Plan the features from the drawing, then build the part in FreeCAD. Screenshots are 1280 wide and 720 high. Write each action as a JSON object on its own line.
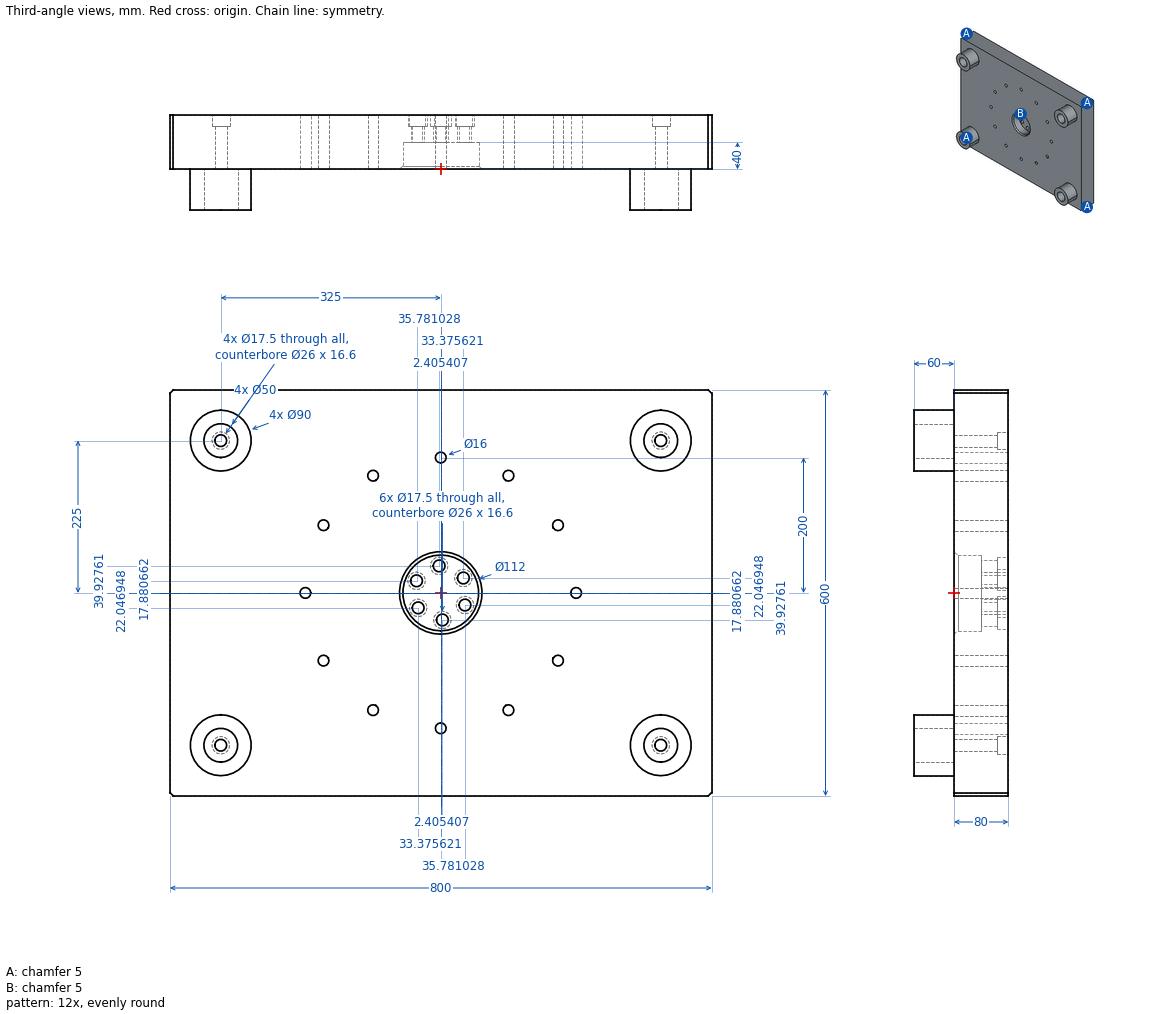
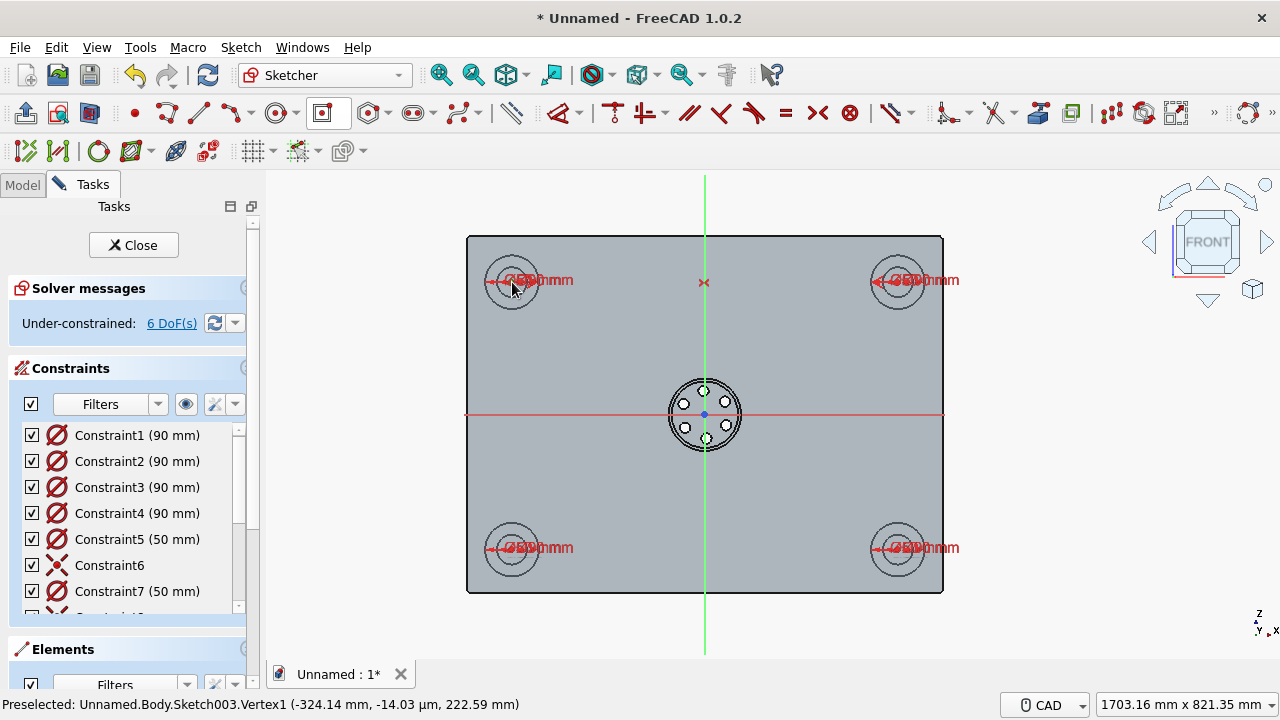
{"action": "left_click", "coordinate": [512, 550]}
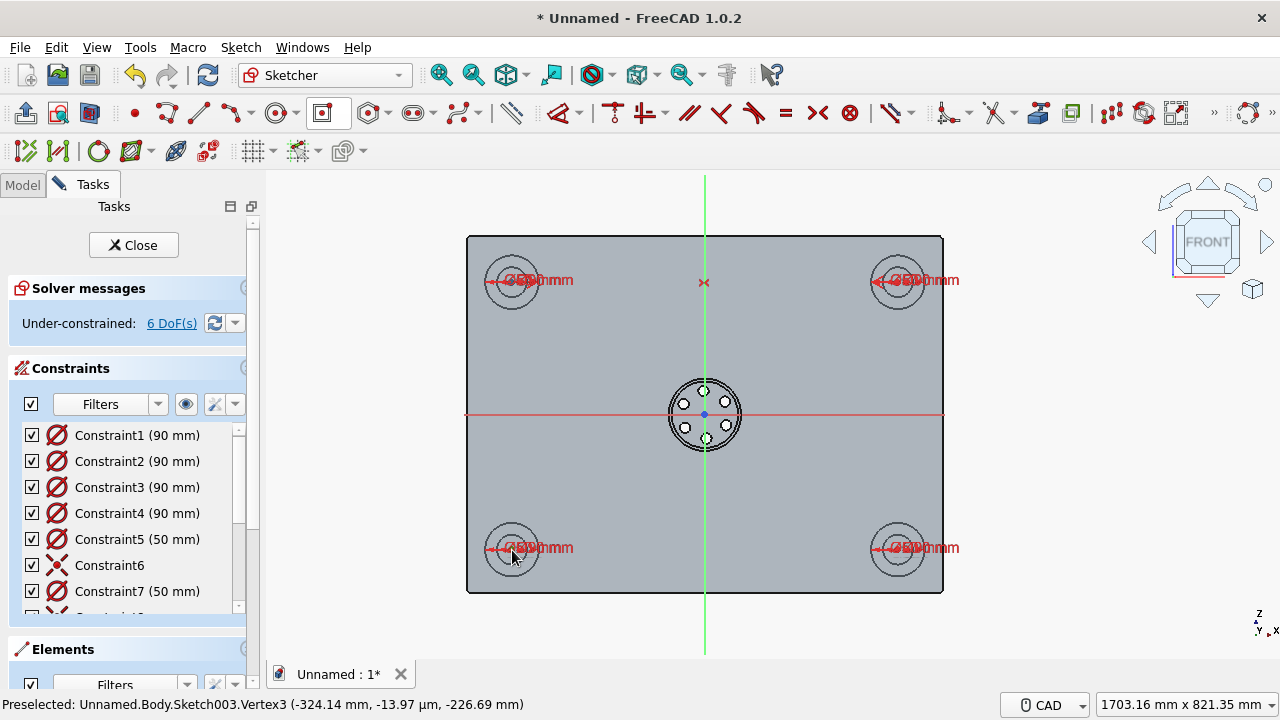
{"action": "left_click", "coordinate": [470, 415]}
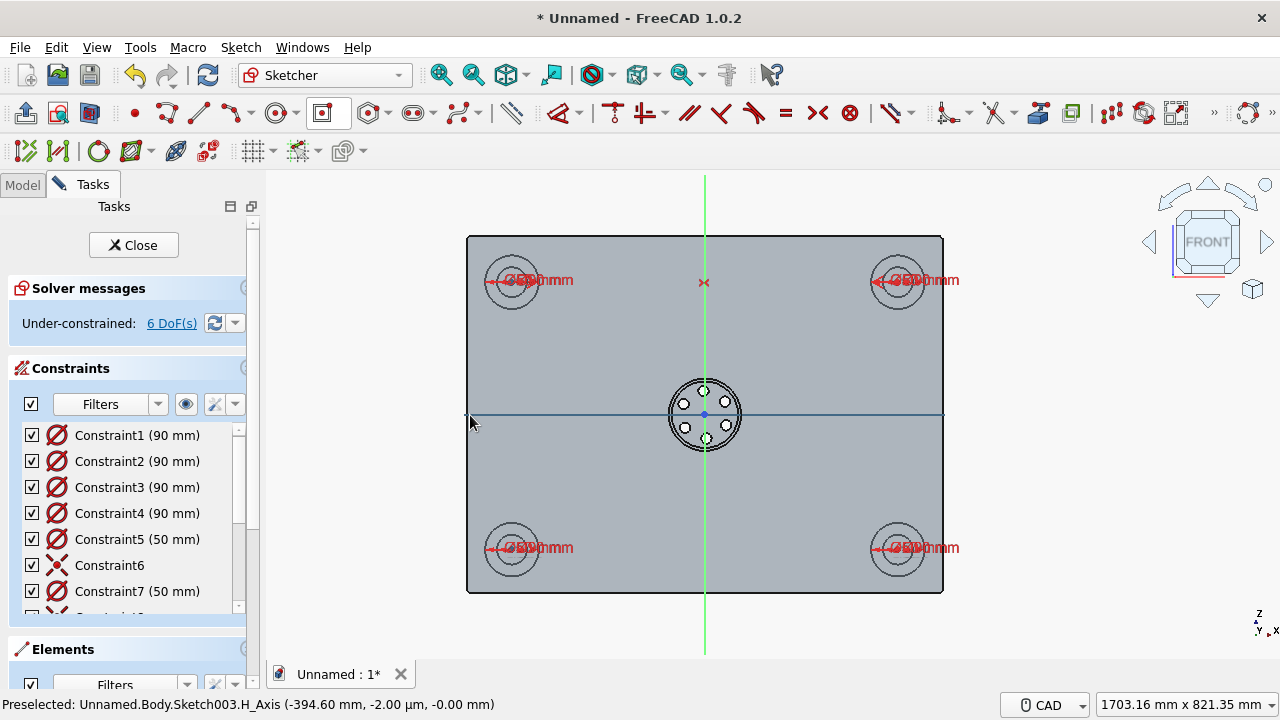
{"action": "key", "text": "s"}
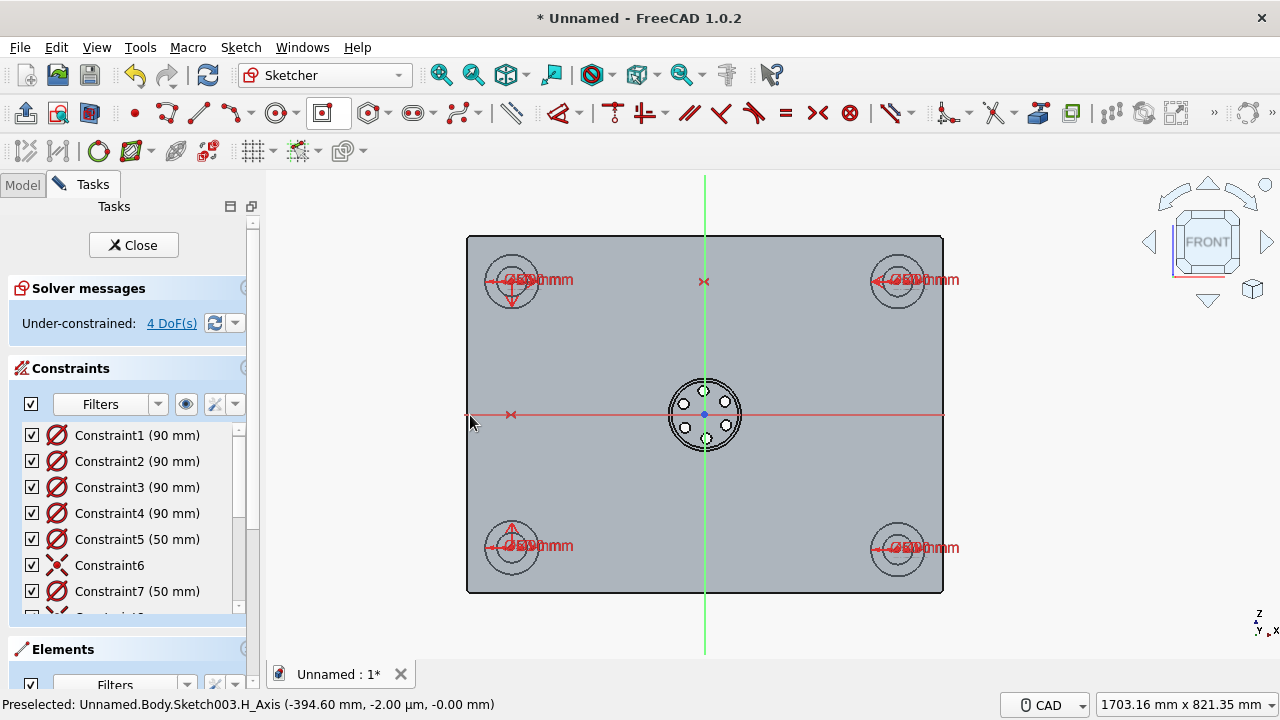
{"action": "left_click", "coordinate": [898, 282]}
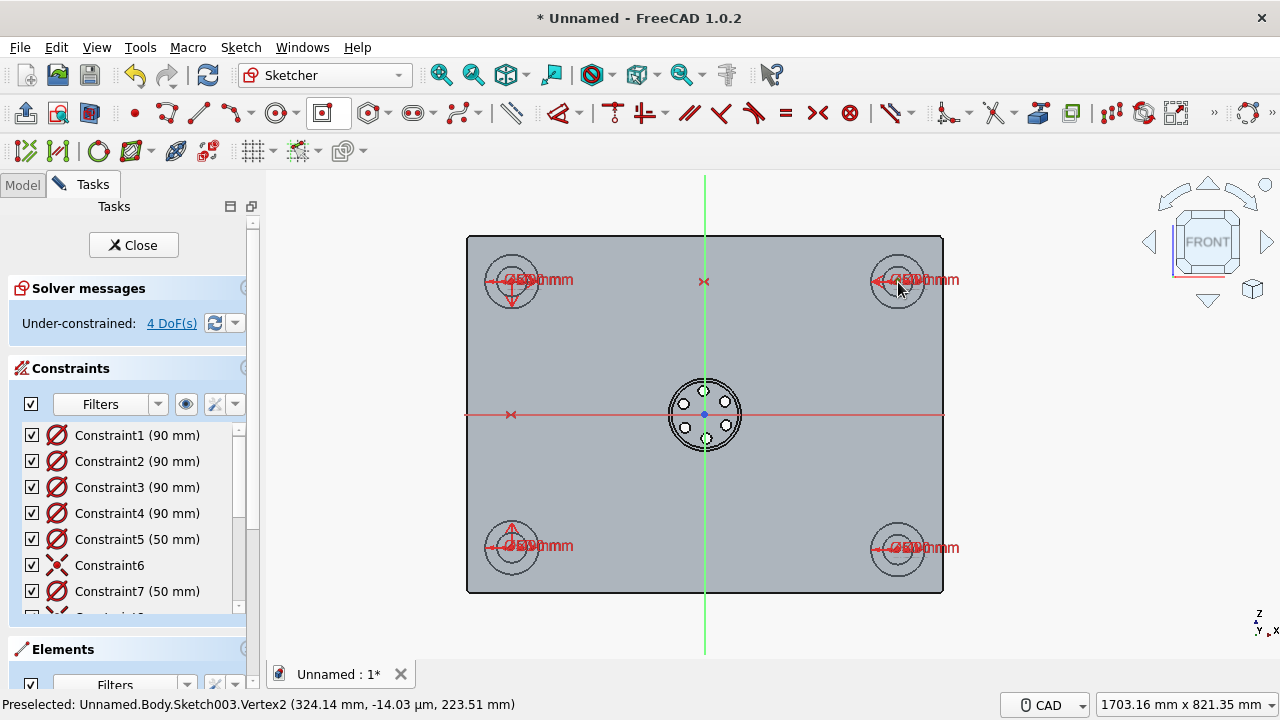
{"action": "left_click", "coordinate": [898, 550]}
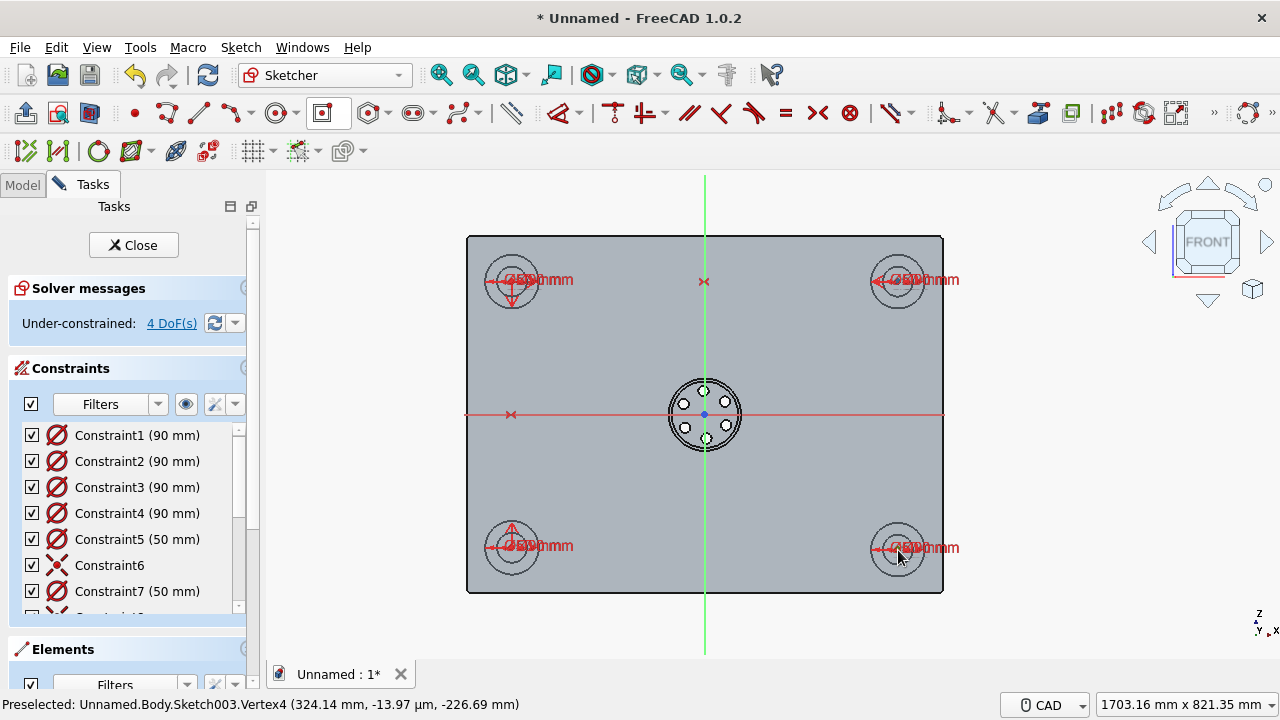
{"action": "left_click", "coordinate": [470, 415]}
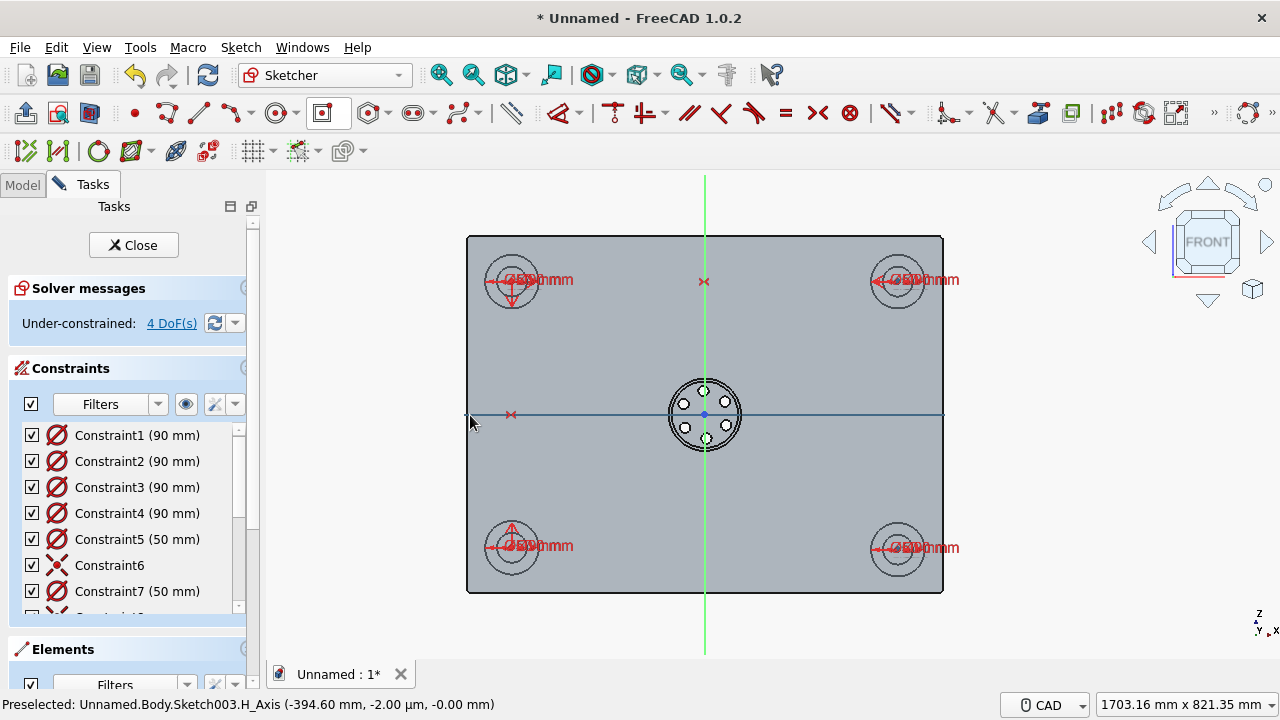
{"action": "key", "text": "s"}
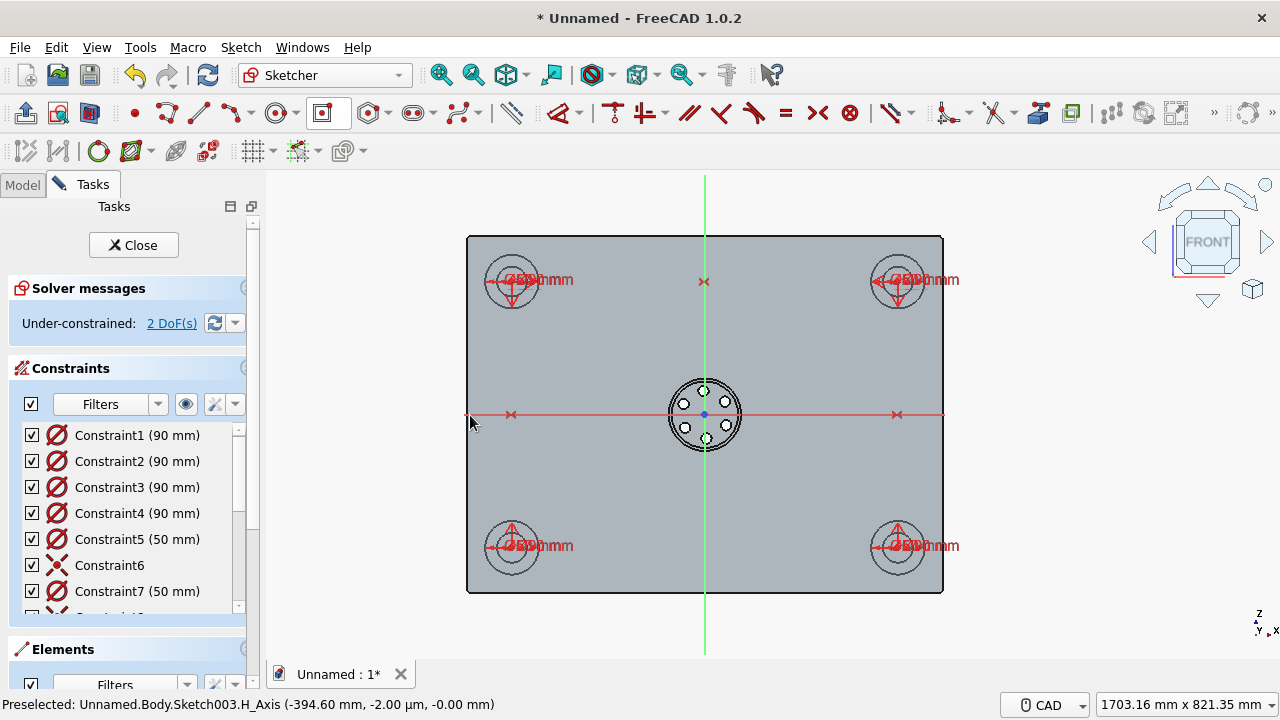
{"action": "left_click", "coordinate": [512, 282]}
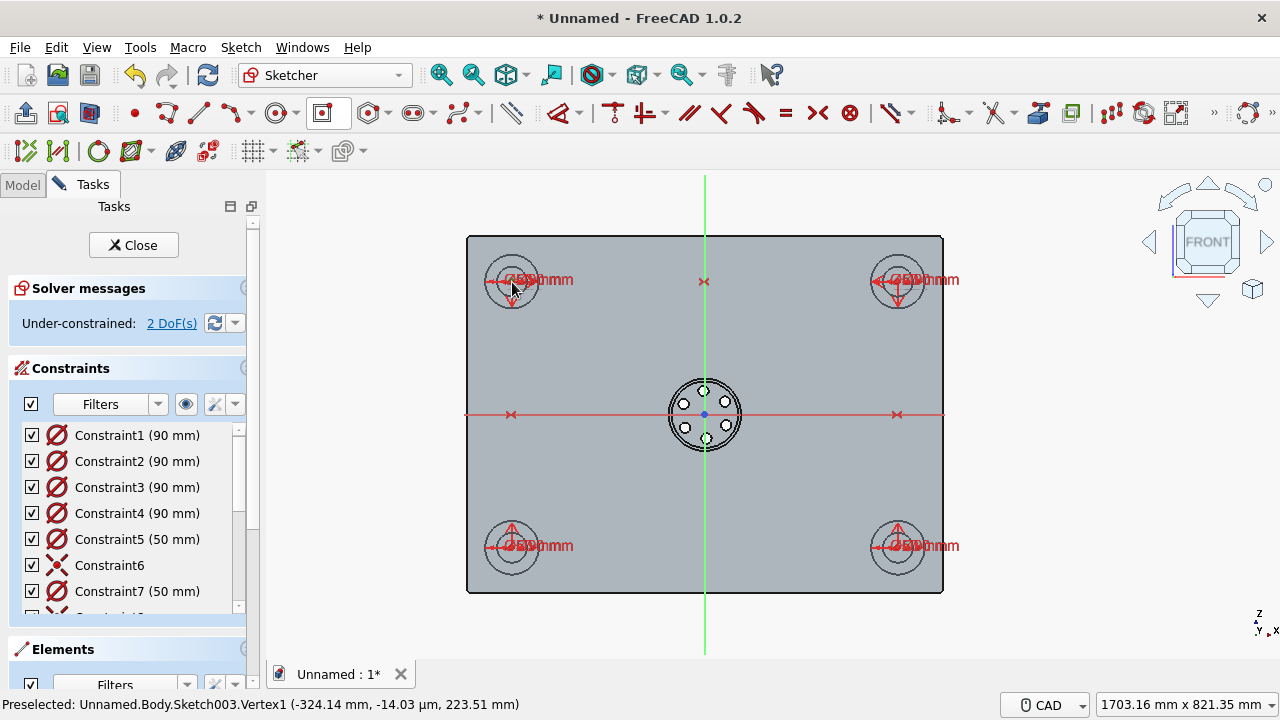
{"action": "key", "text": "l"}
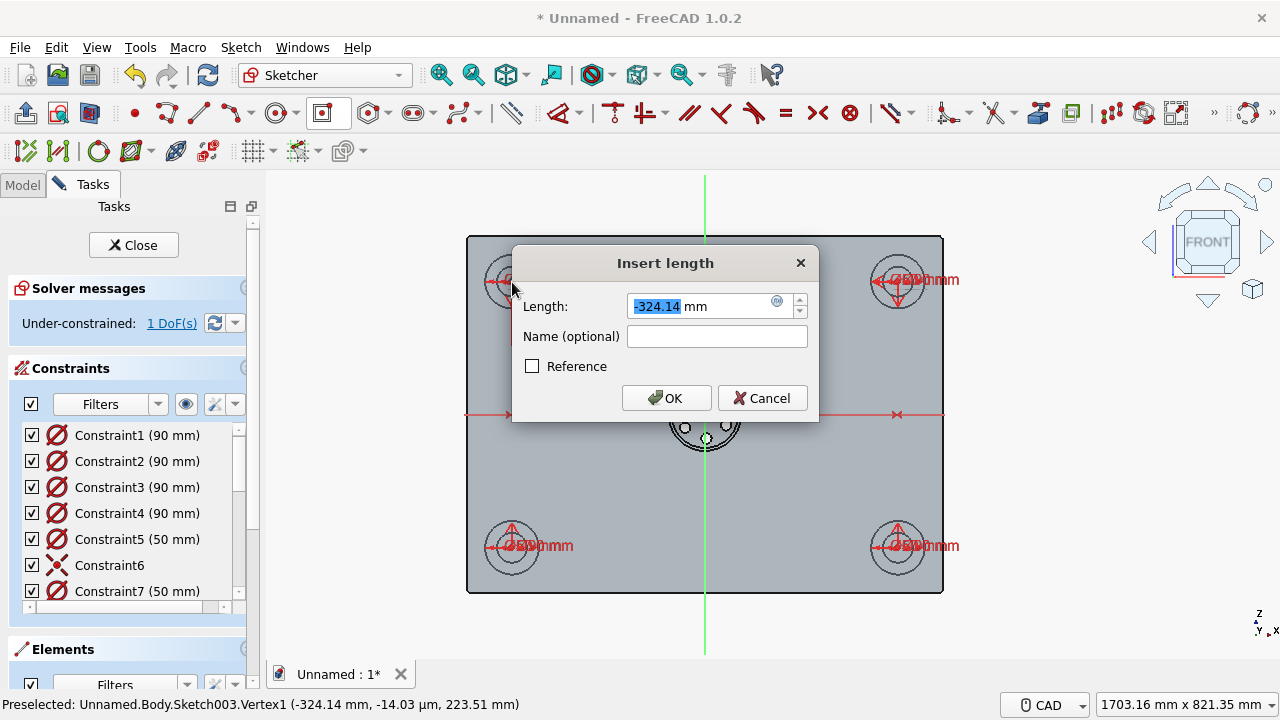
{"action": "type", "text": "-325"}
{"action": "key", "text": "Return"}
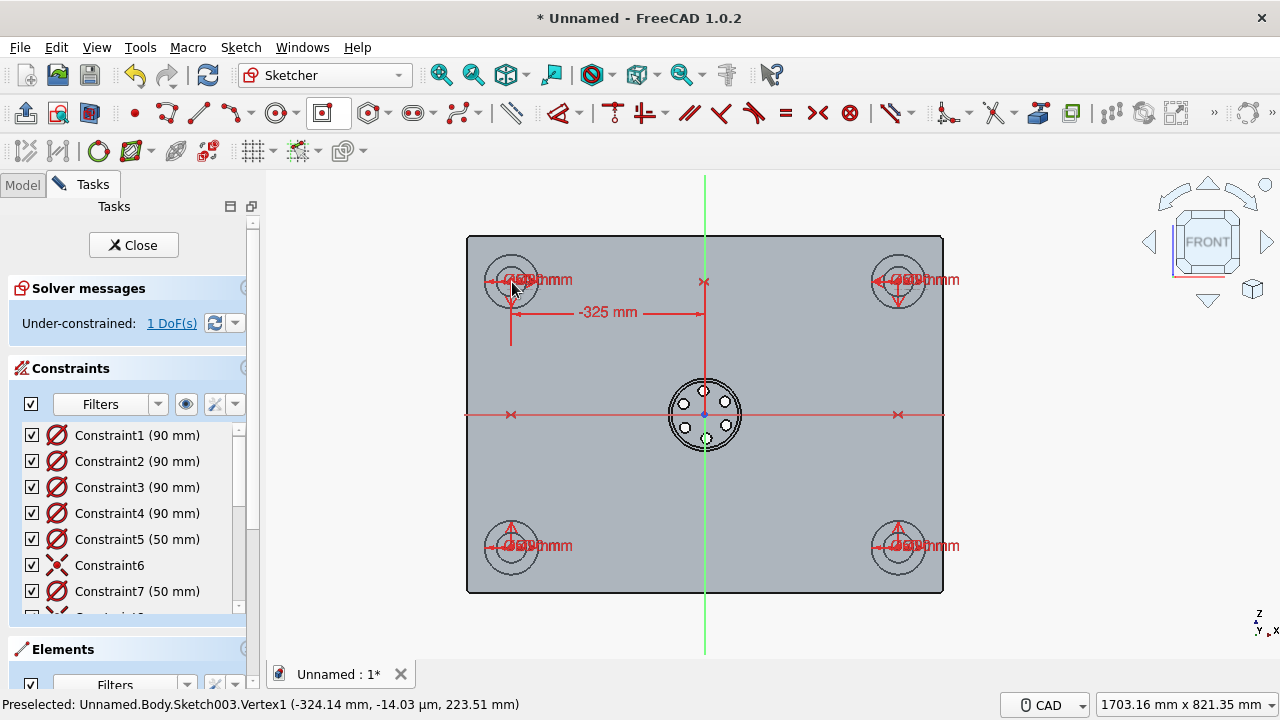
{"action": "left_click", "coordinate": [511, 282]}